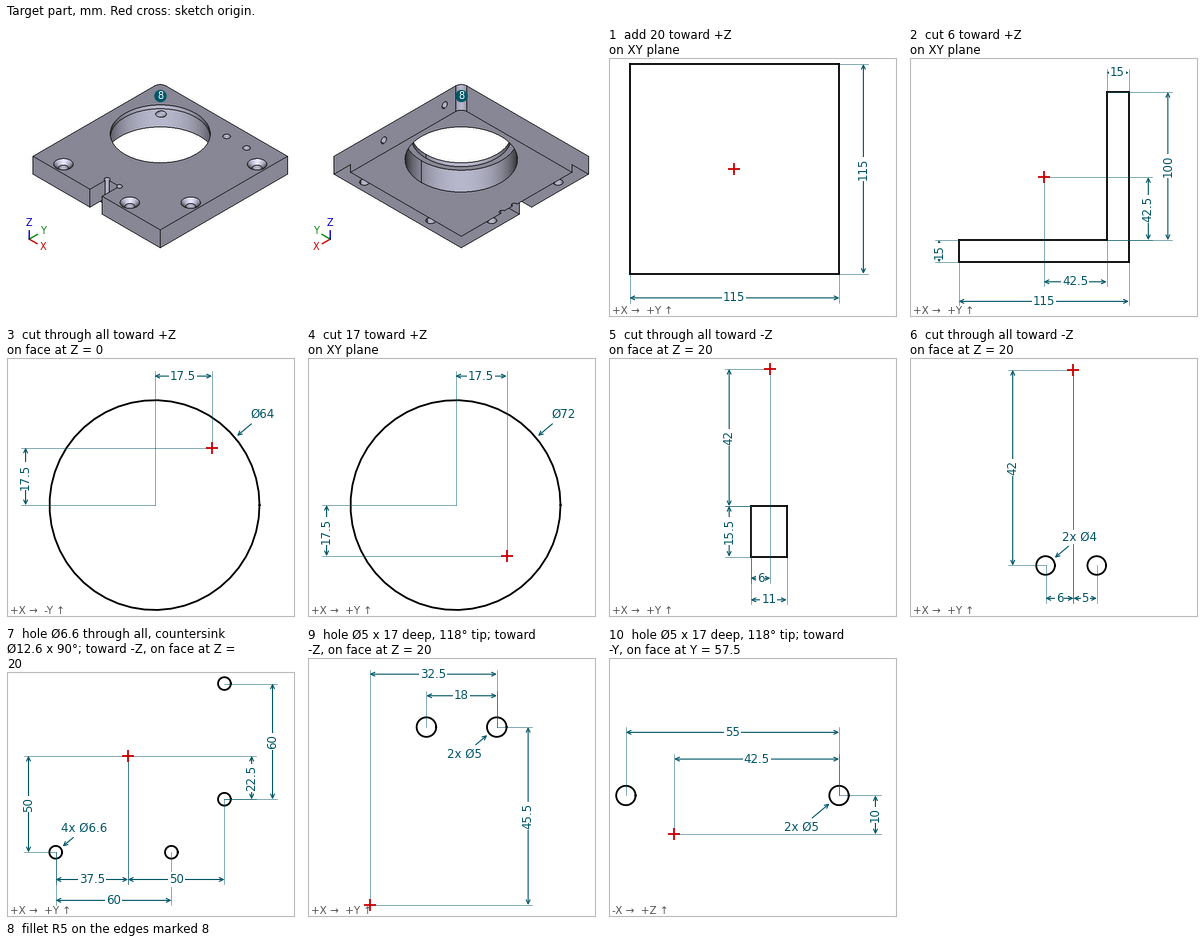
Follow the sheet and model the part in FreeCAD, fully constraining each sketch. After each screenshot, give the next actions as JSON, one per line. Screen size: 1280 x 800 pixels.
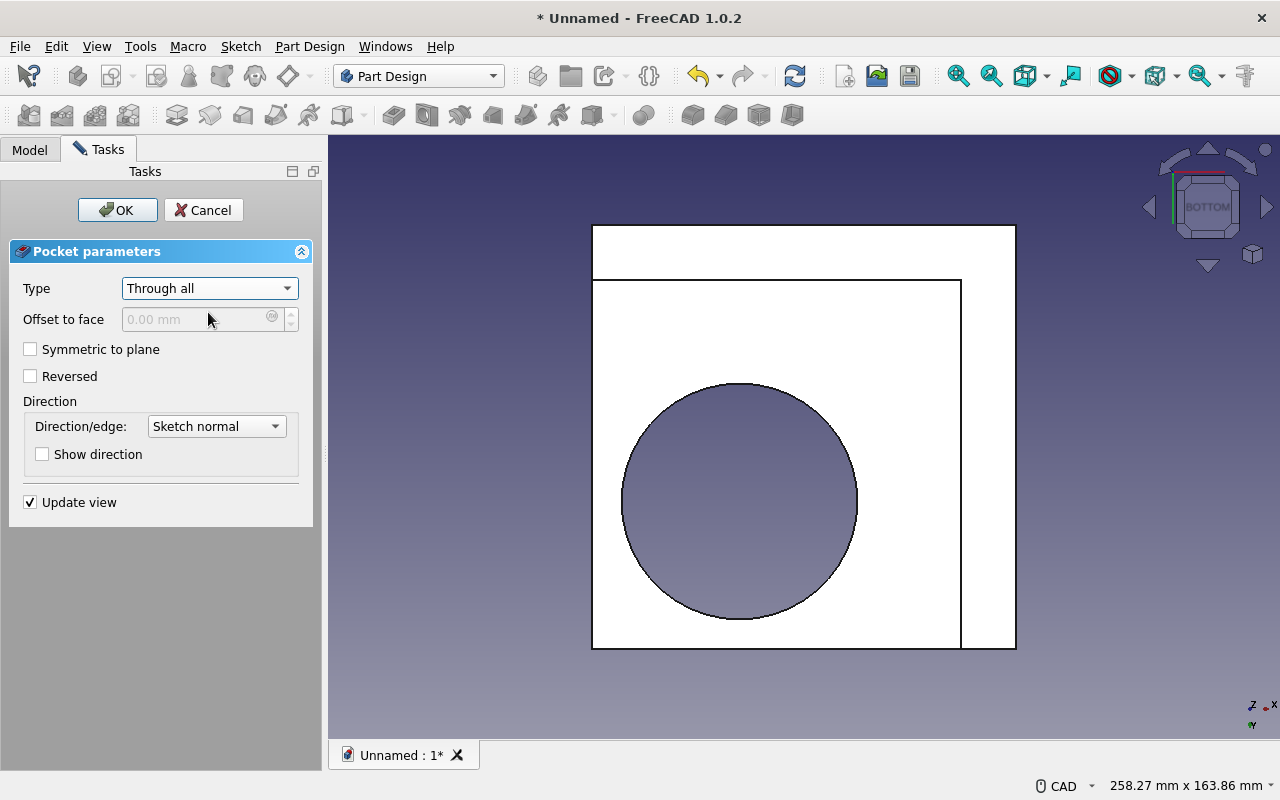
{"action": "left_click", "coordinate": [118, 210]}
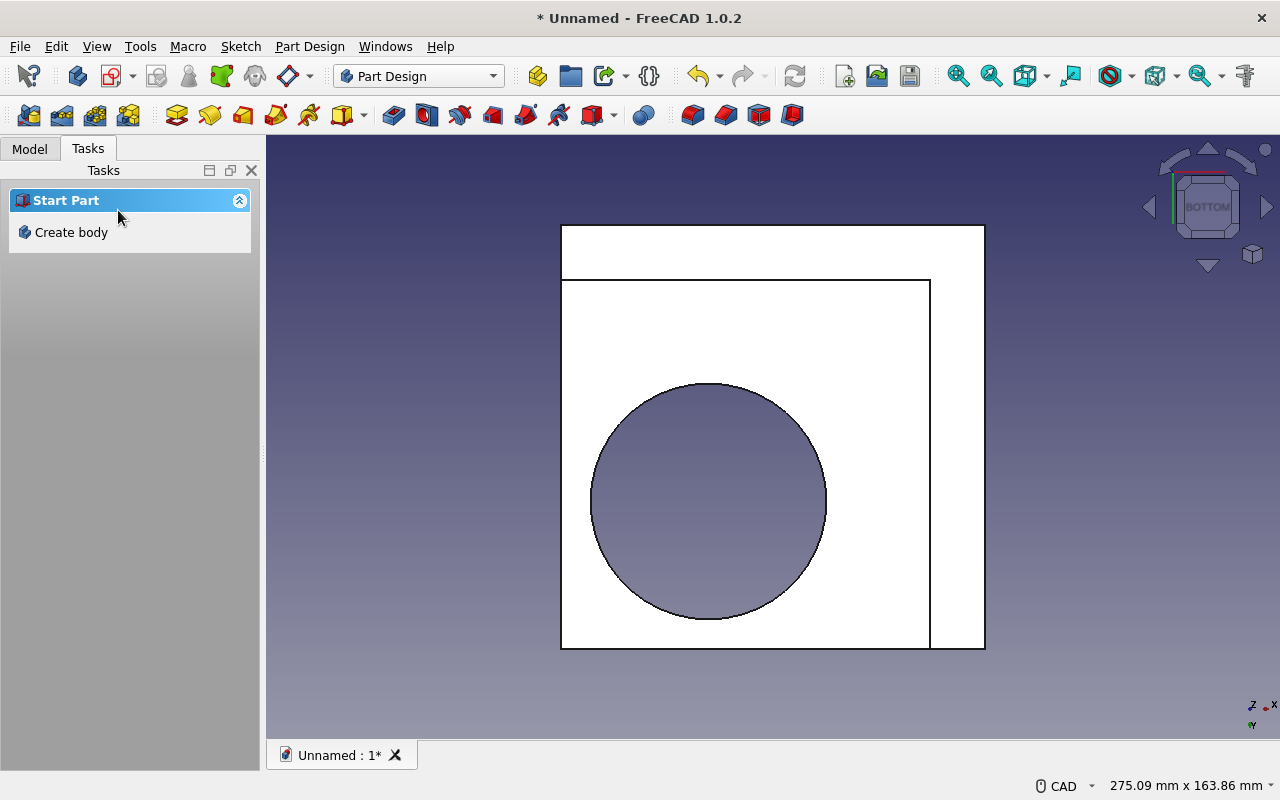
{"action": "left_click", "coordinate": [110, 76]}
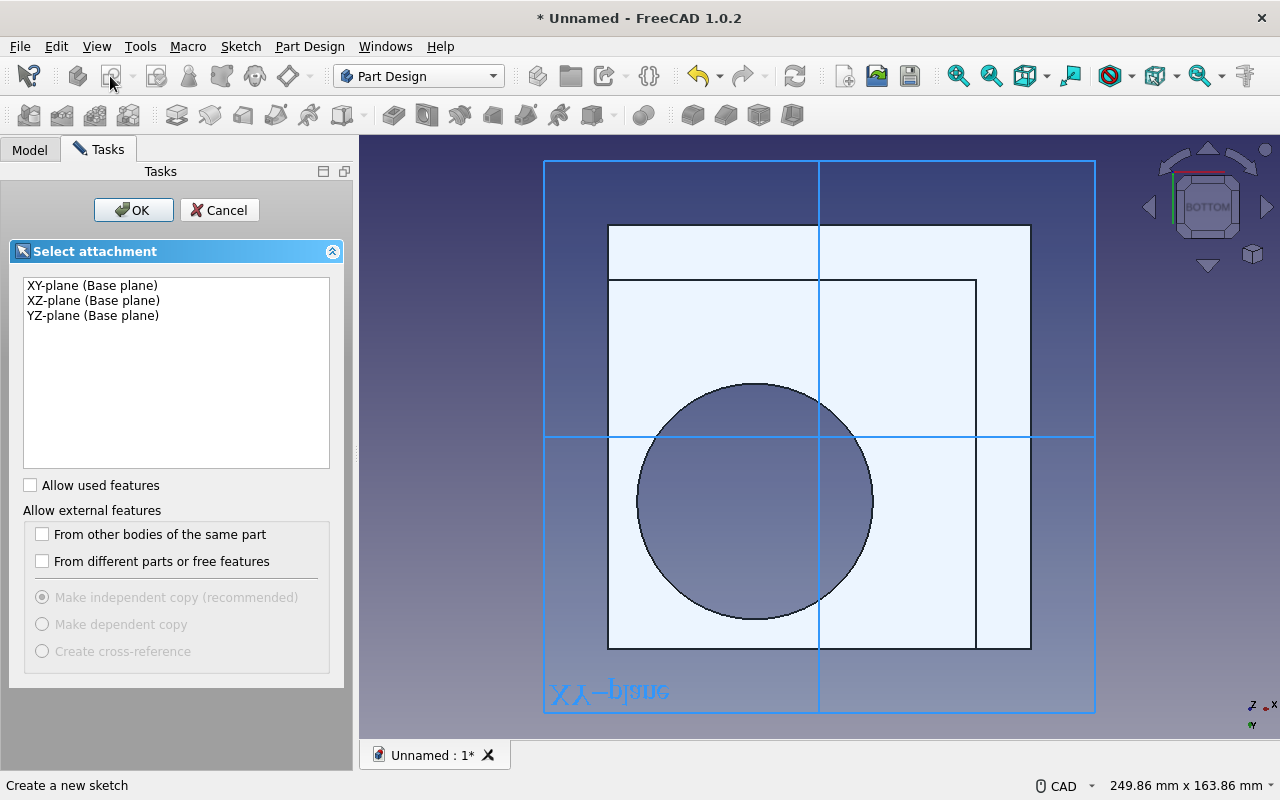
{"action": "left_click", "coordinate": [84, 286]}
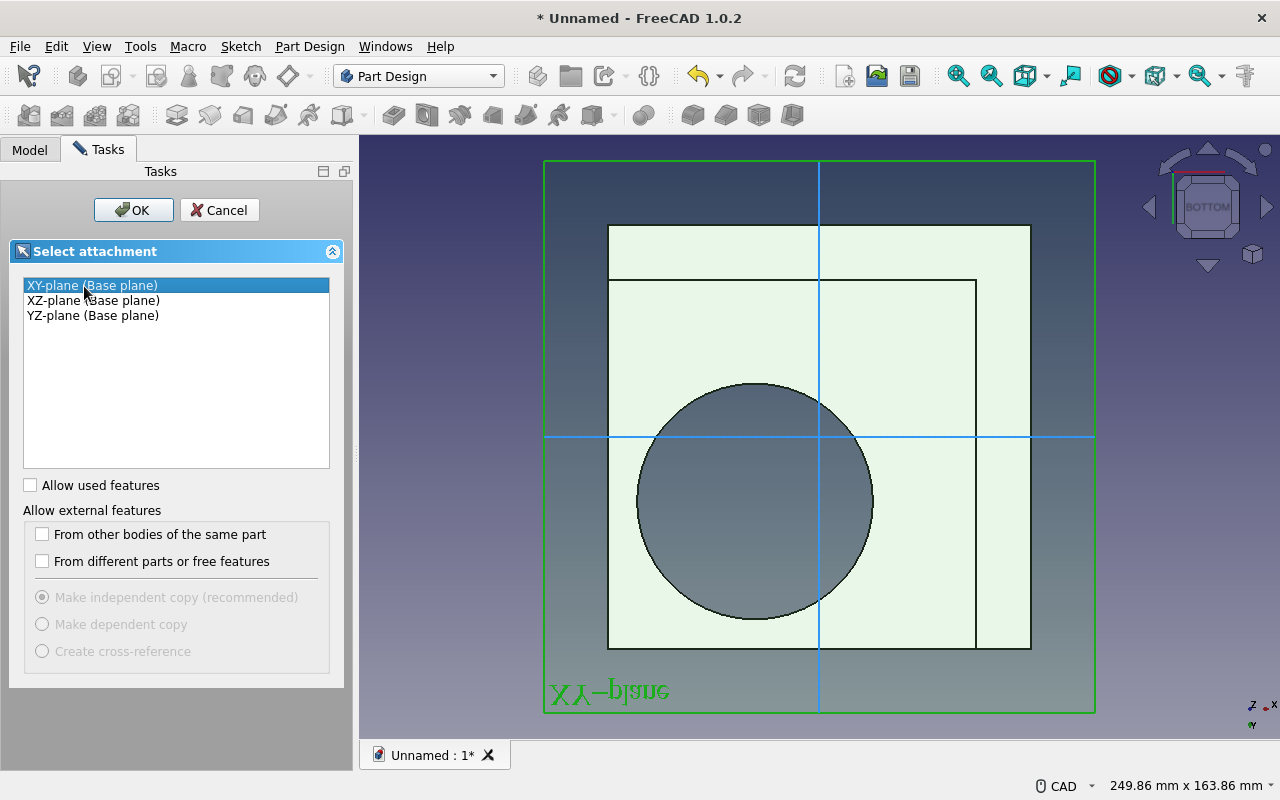
{"action": "left_click", "coordinate": [134, 210]}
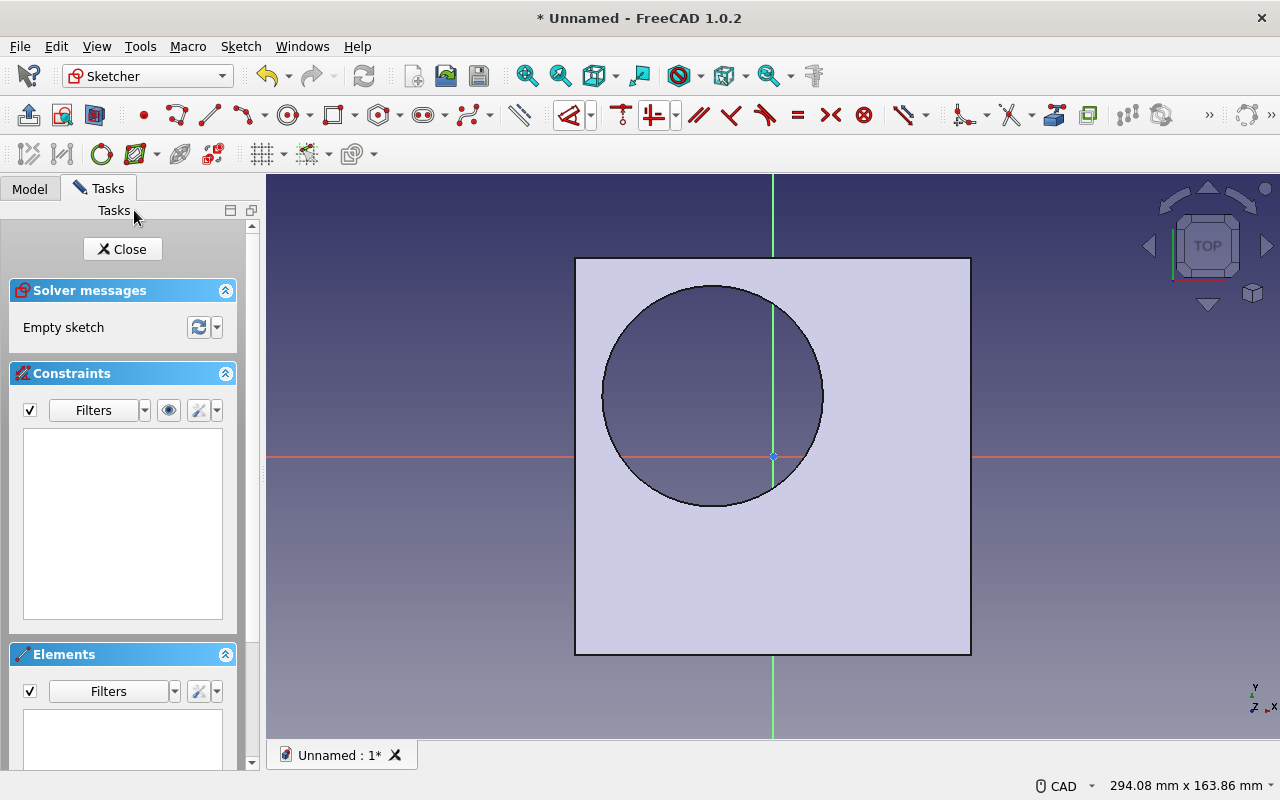
{"action": "key", "text": "q s"}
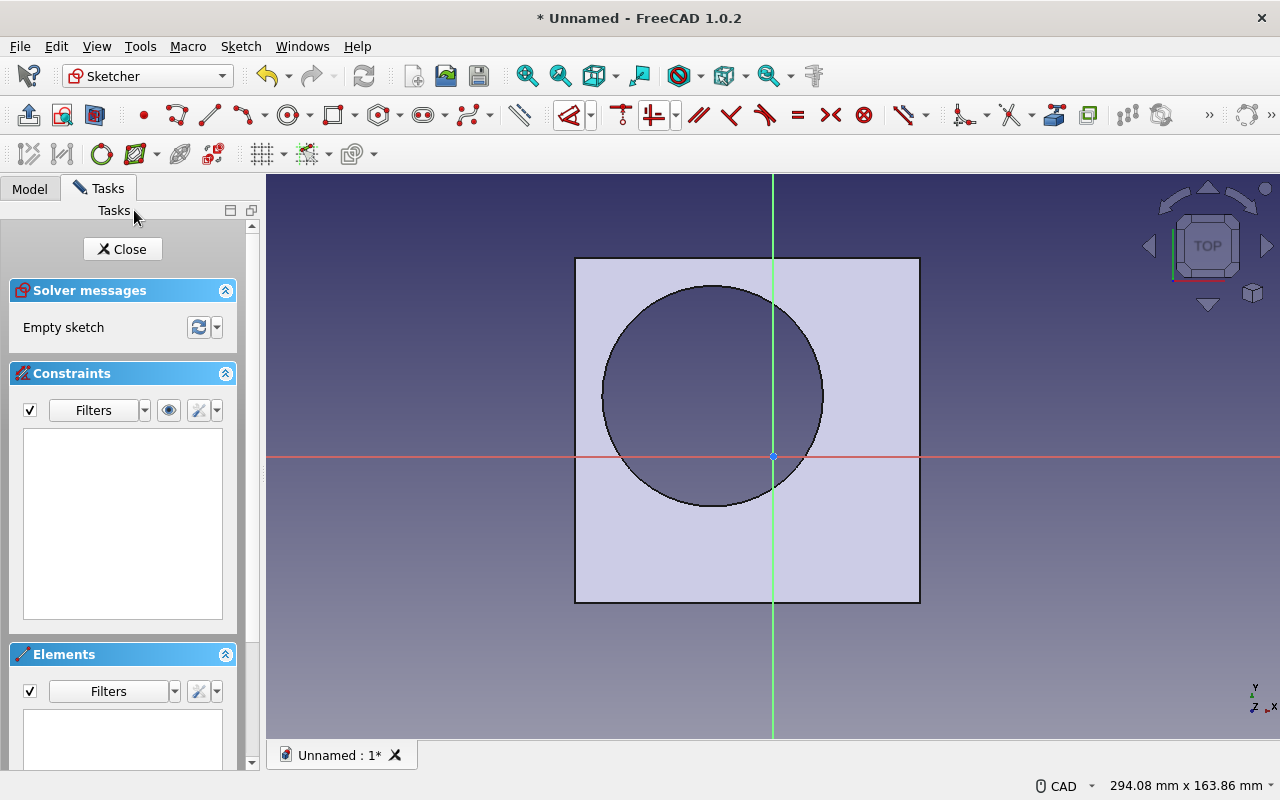
{"action": "scroll", "coordinate": [729, 273], "scroll_direction": "up", "scroll_amount": 2}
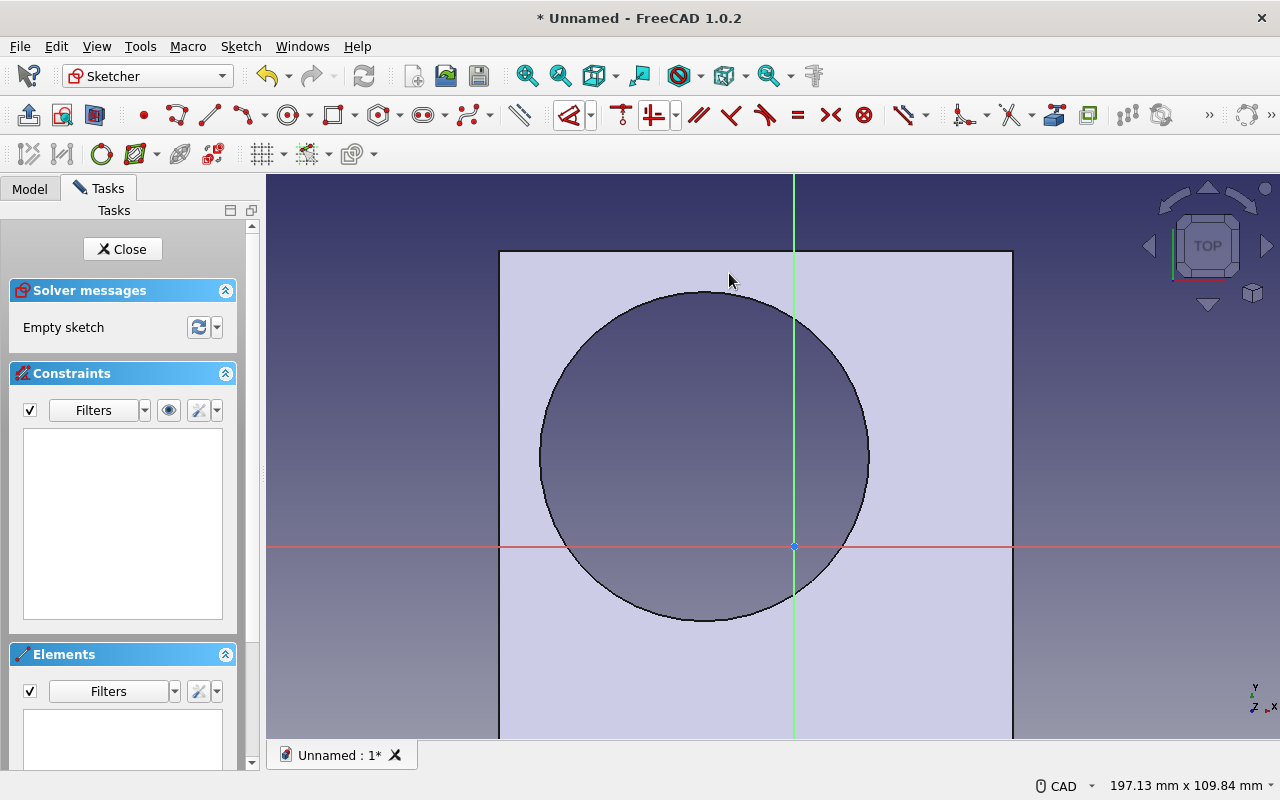
{"action": "key", "text": "g c"}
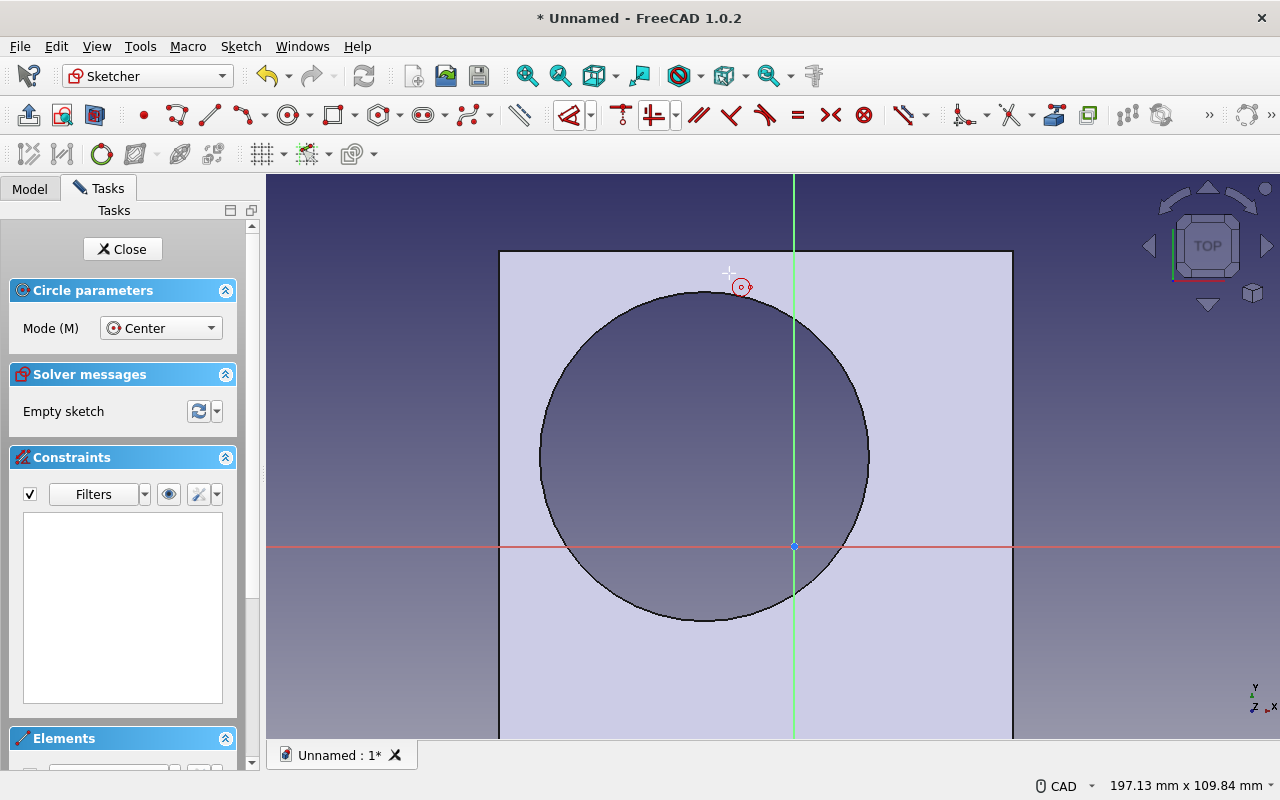
{"action": "left_click", "coordinate": [704, 457]}
{"action": "left_click", "coordinate": [835, 326]}
{"action": "key", "text": "Escape"}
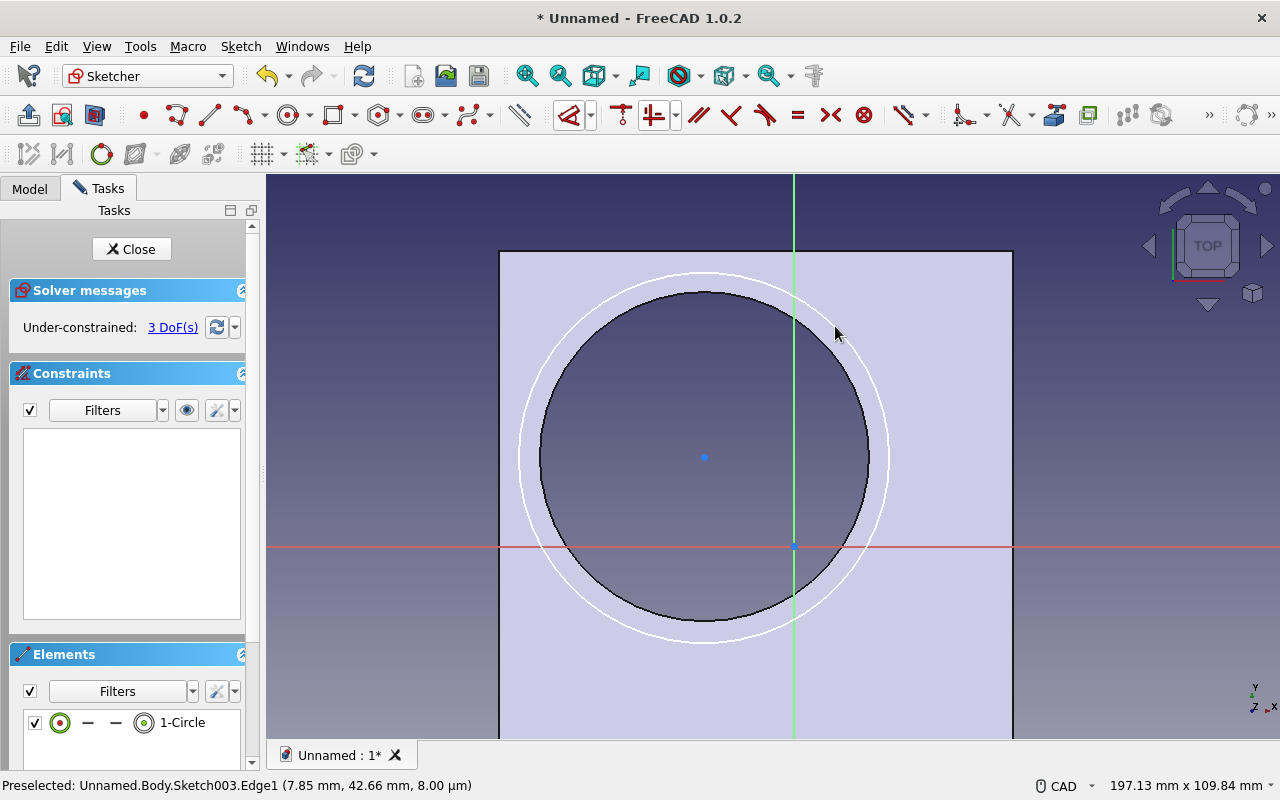
{"action": "left_click", "coordinate": [835, 327]}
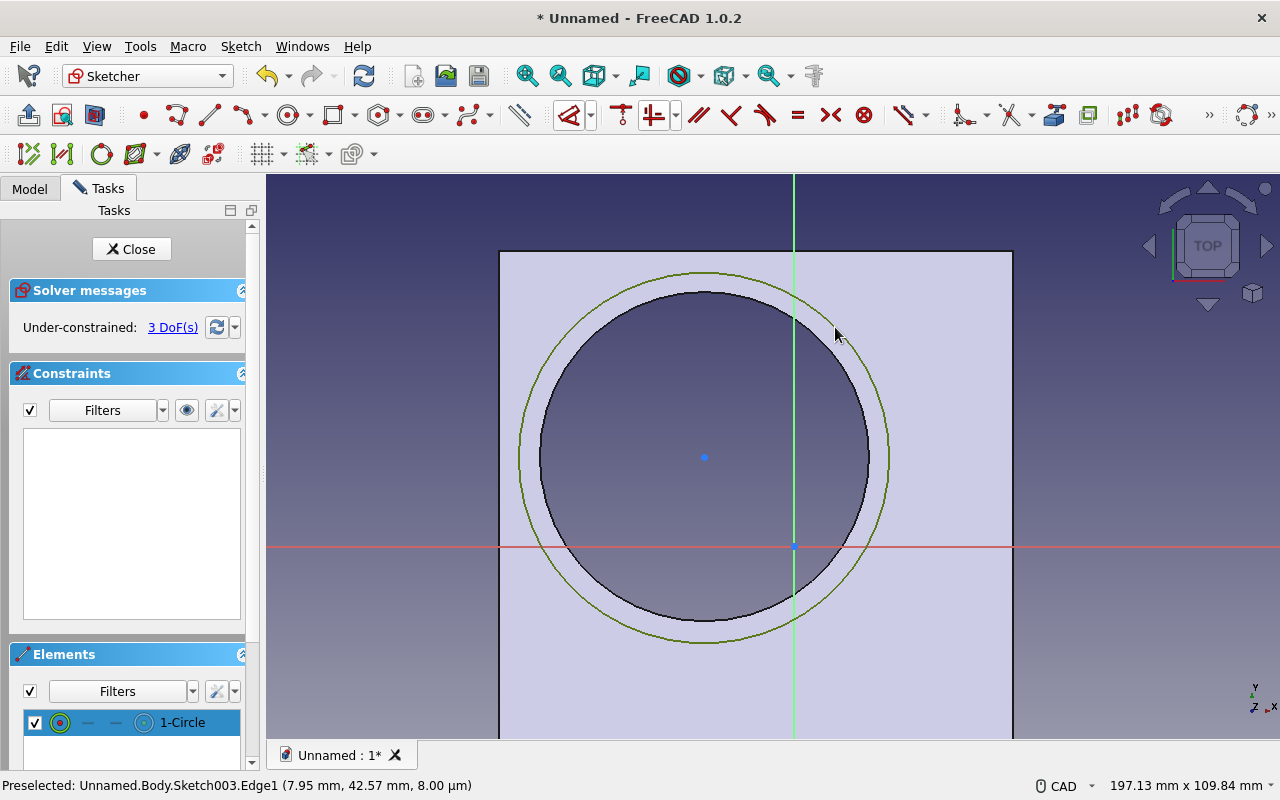
{"action": "key", "text": "k o"}